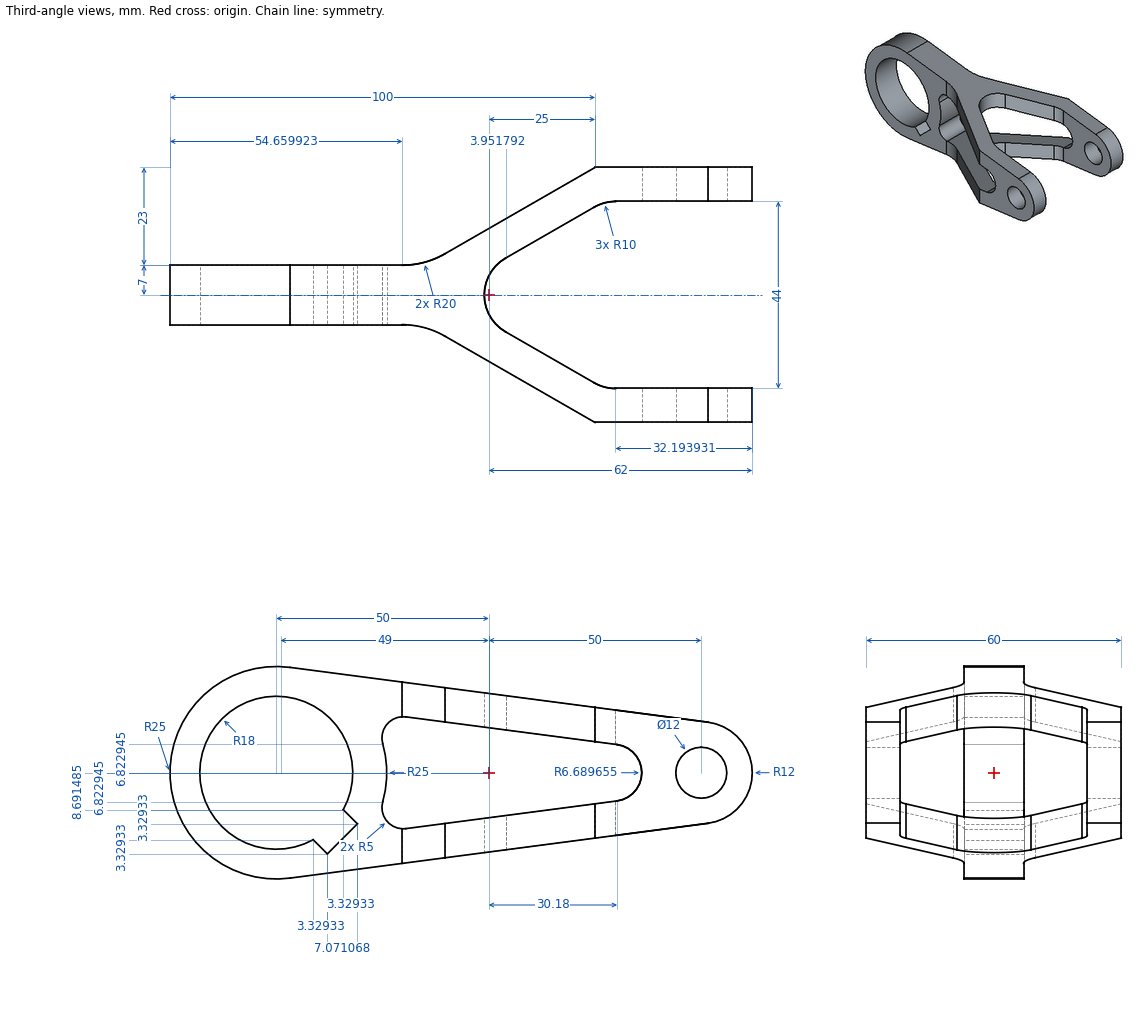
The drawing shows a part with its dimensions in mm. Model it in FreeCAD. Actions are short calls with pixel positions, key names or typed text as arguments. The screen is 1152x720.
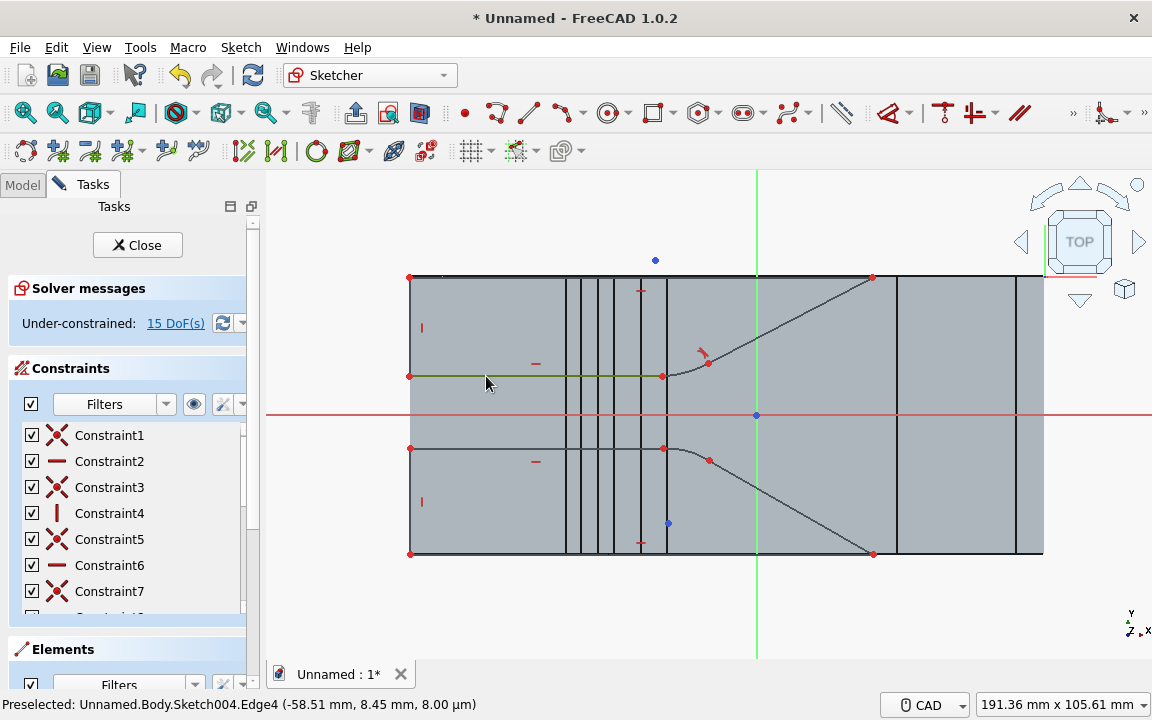
click(677, 374)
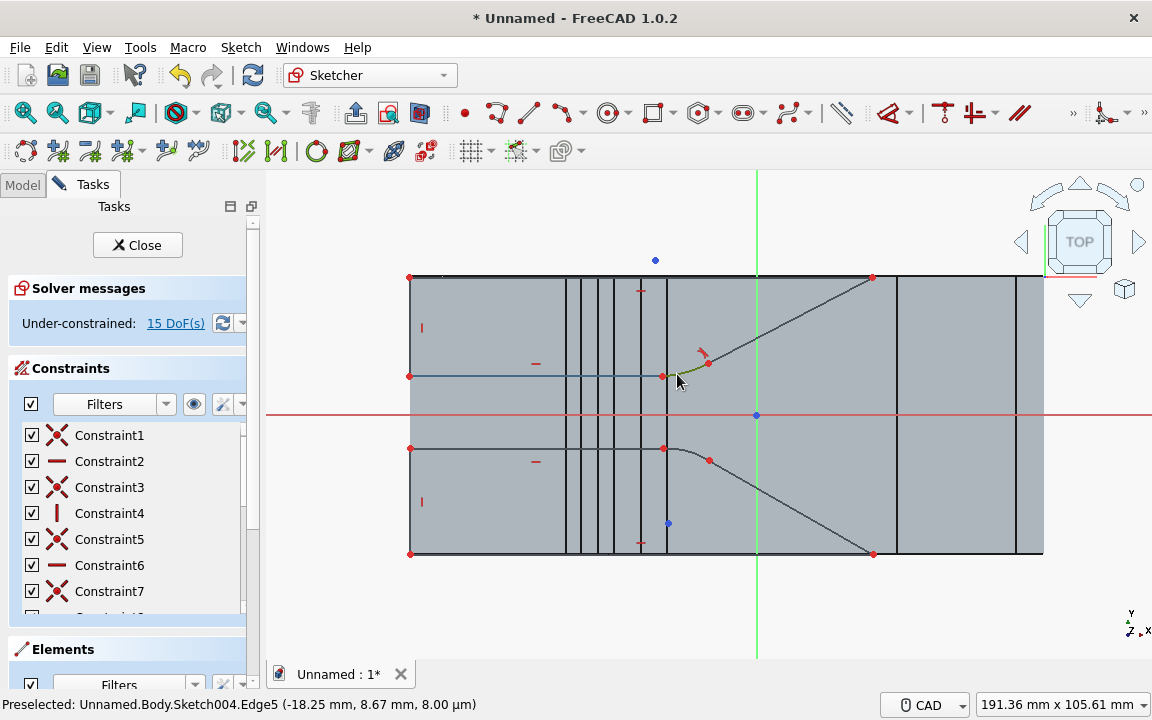
key(t)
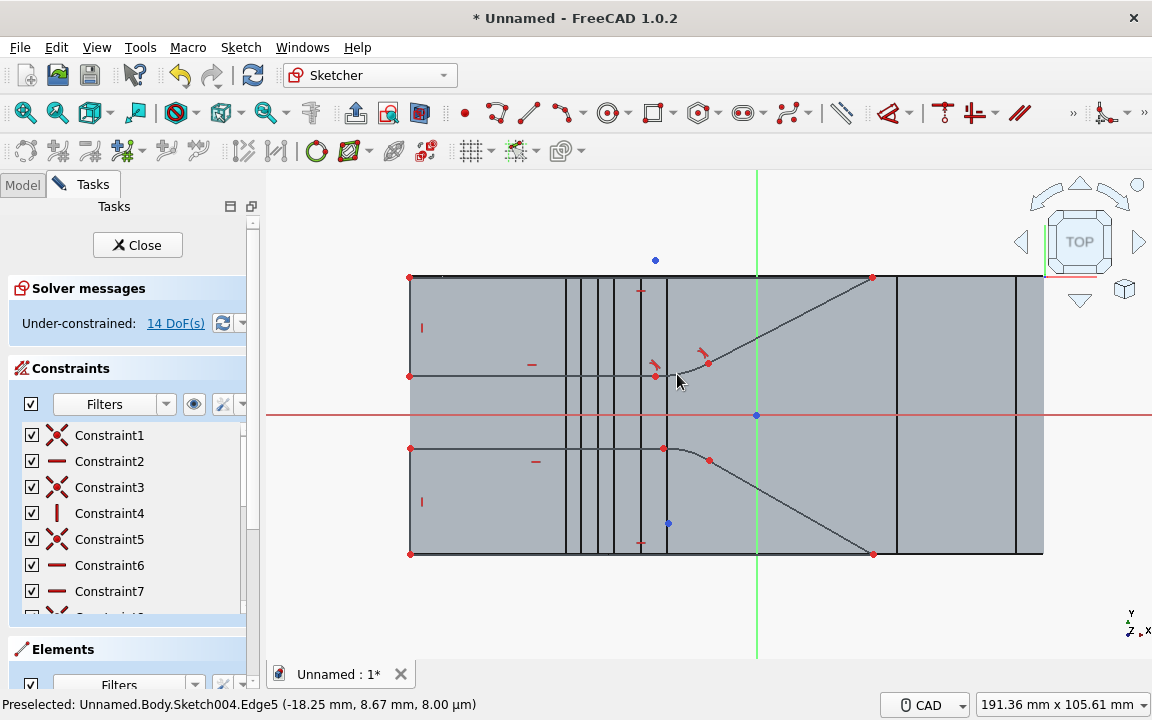
click(587, 449)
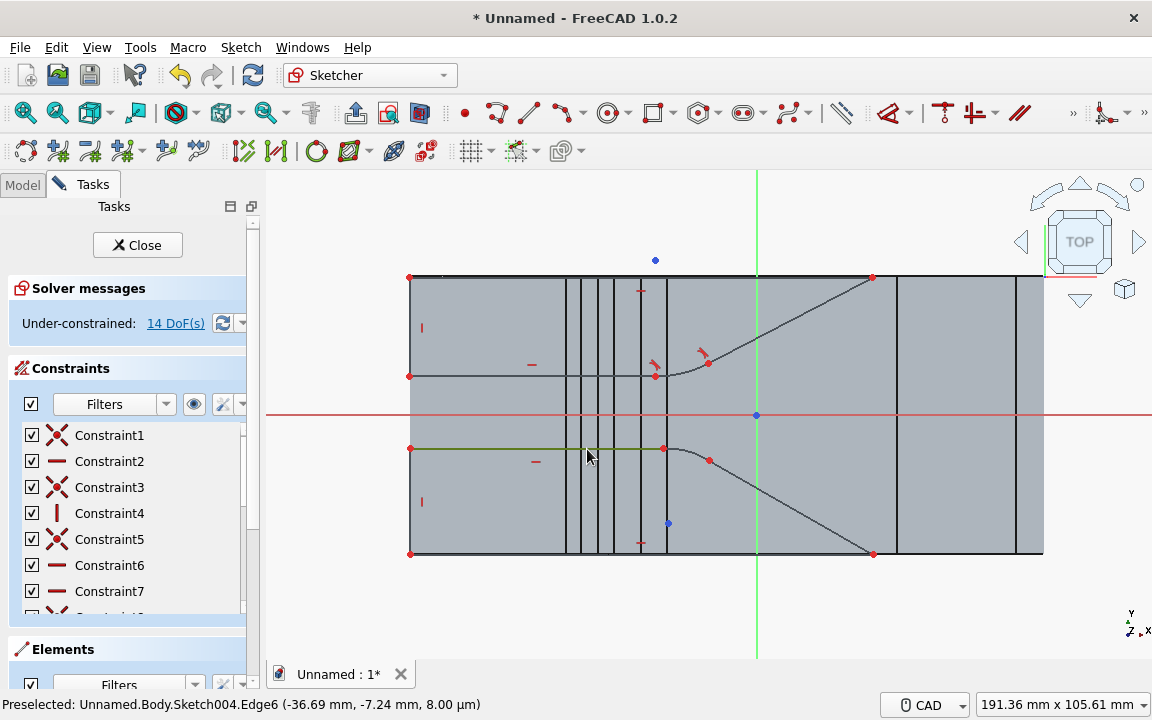
click(696, 454)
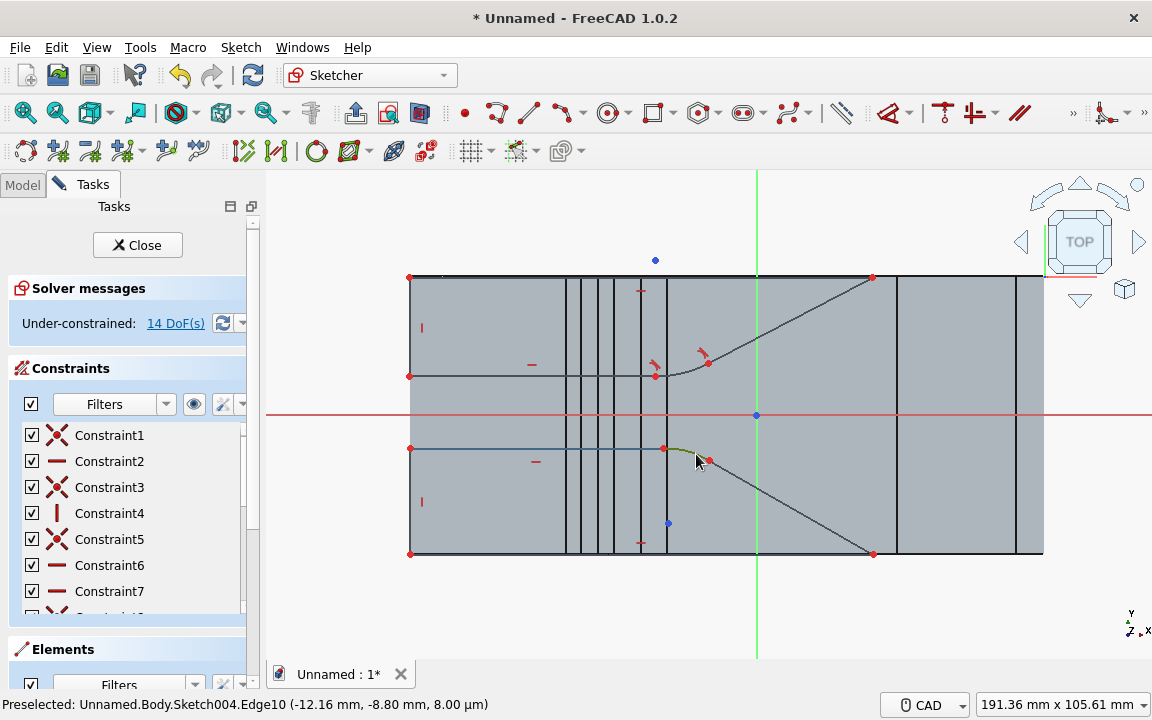
key(t)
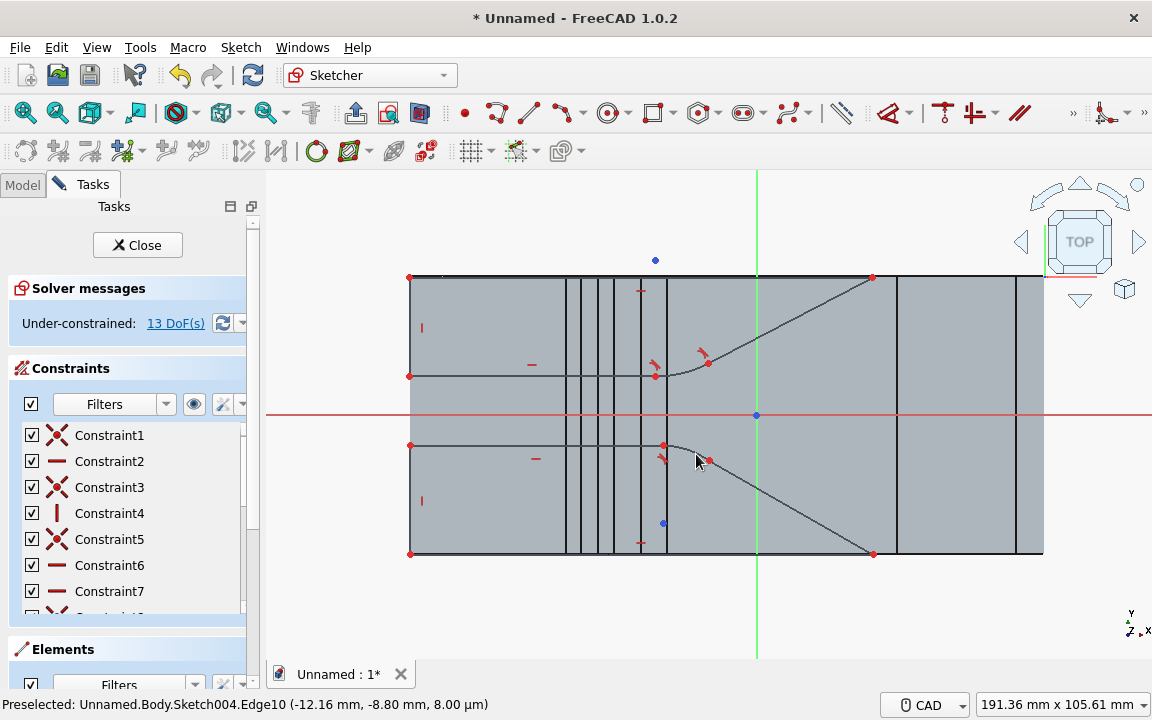
click(824, 527)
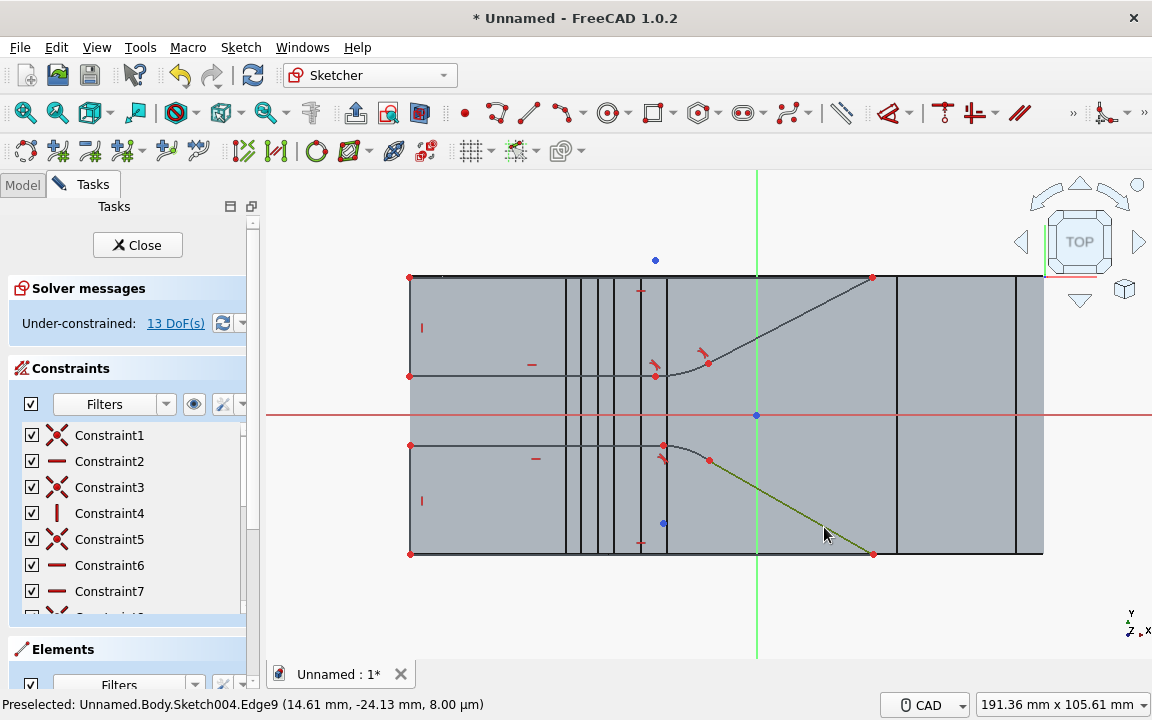
click(696, 453)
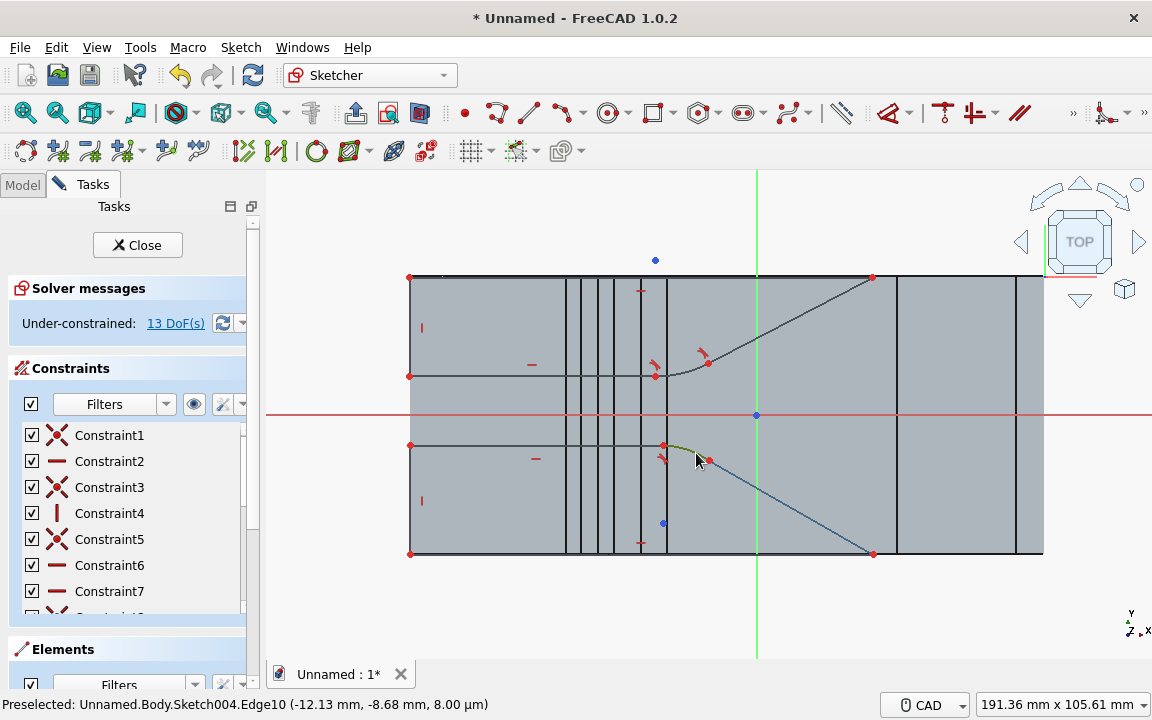
key(t)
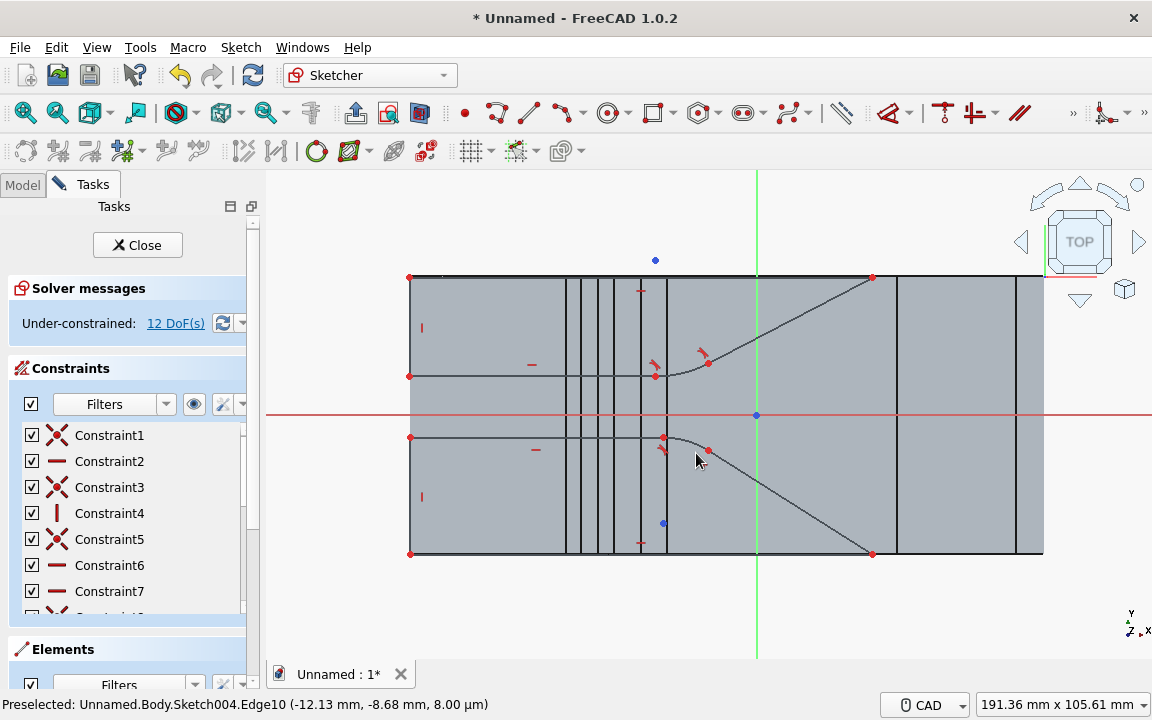
click(672, 375)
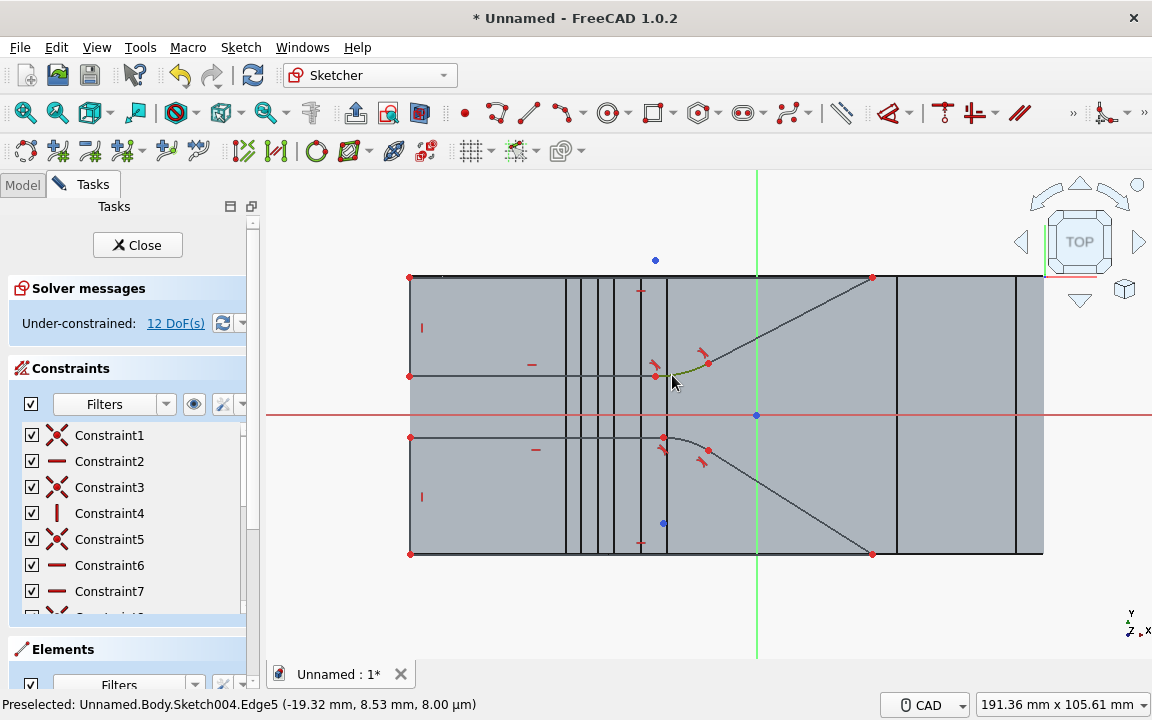
click(696, 444)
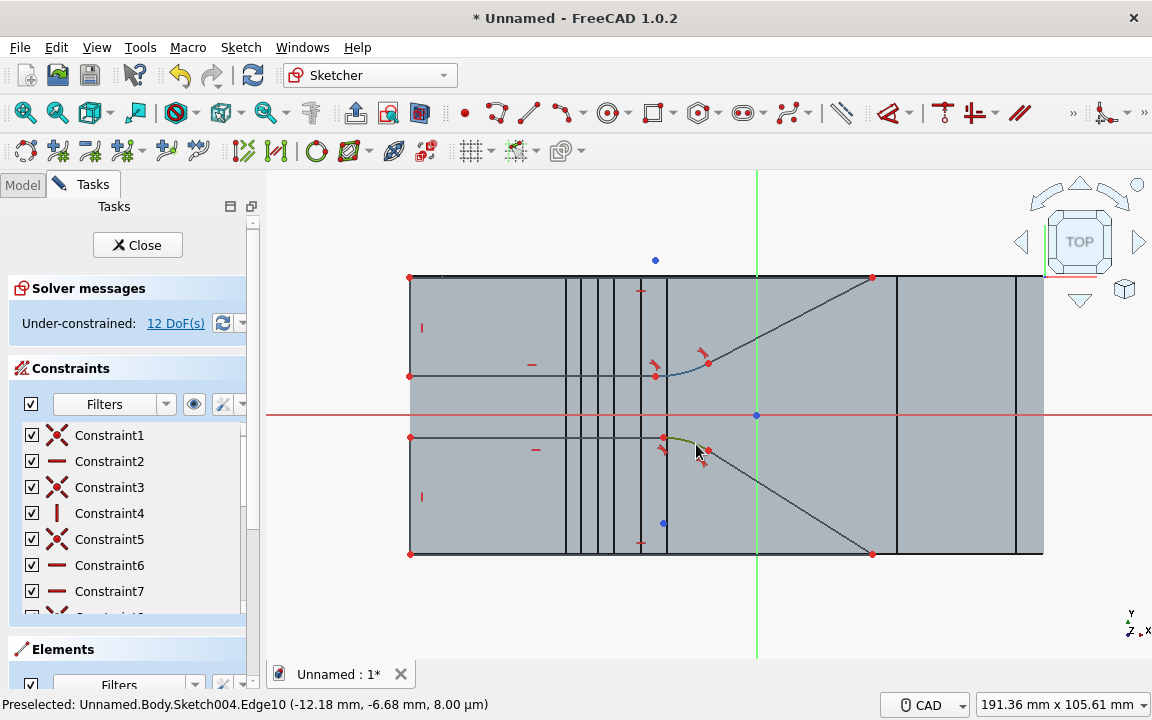
key(e)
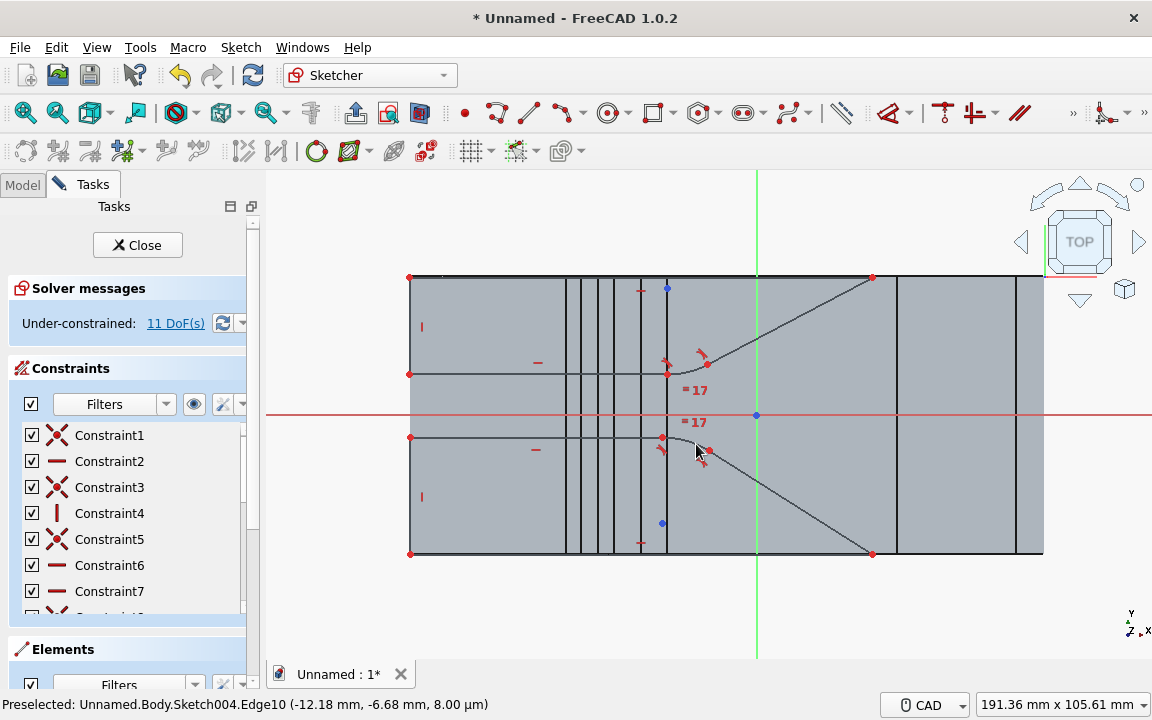
click(668, 288)